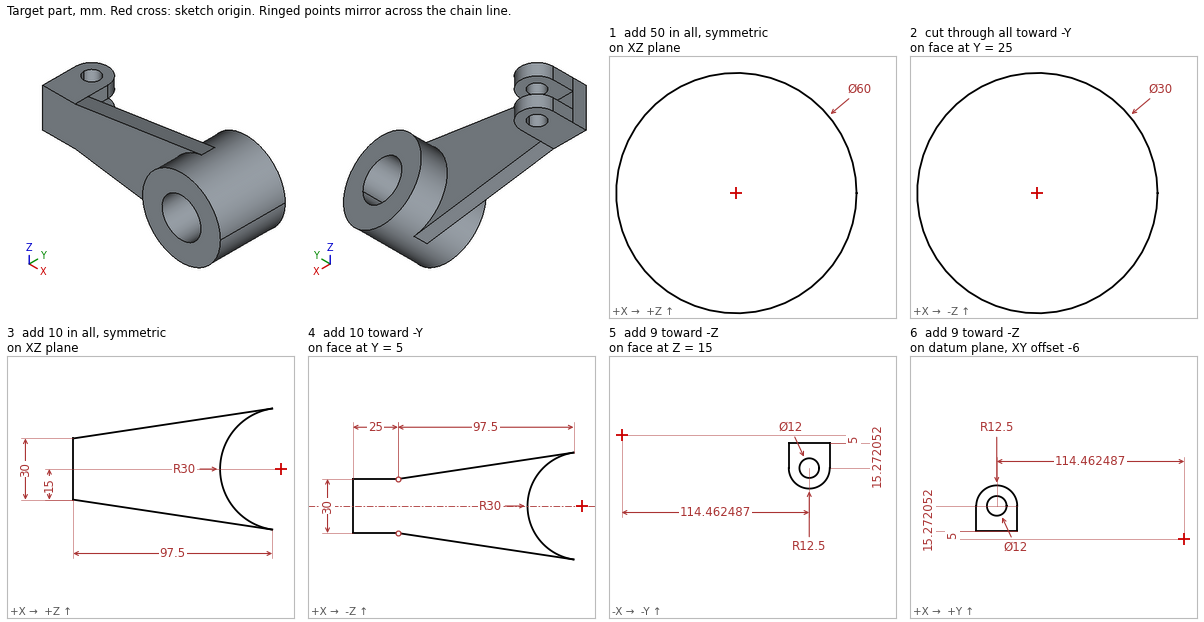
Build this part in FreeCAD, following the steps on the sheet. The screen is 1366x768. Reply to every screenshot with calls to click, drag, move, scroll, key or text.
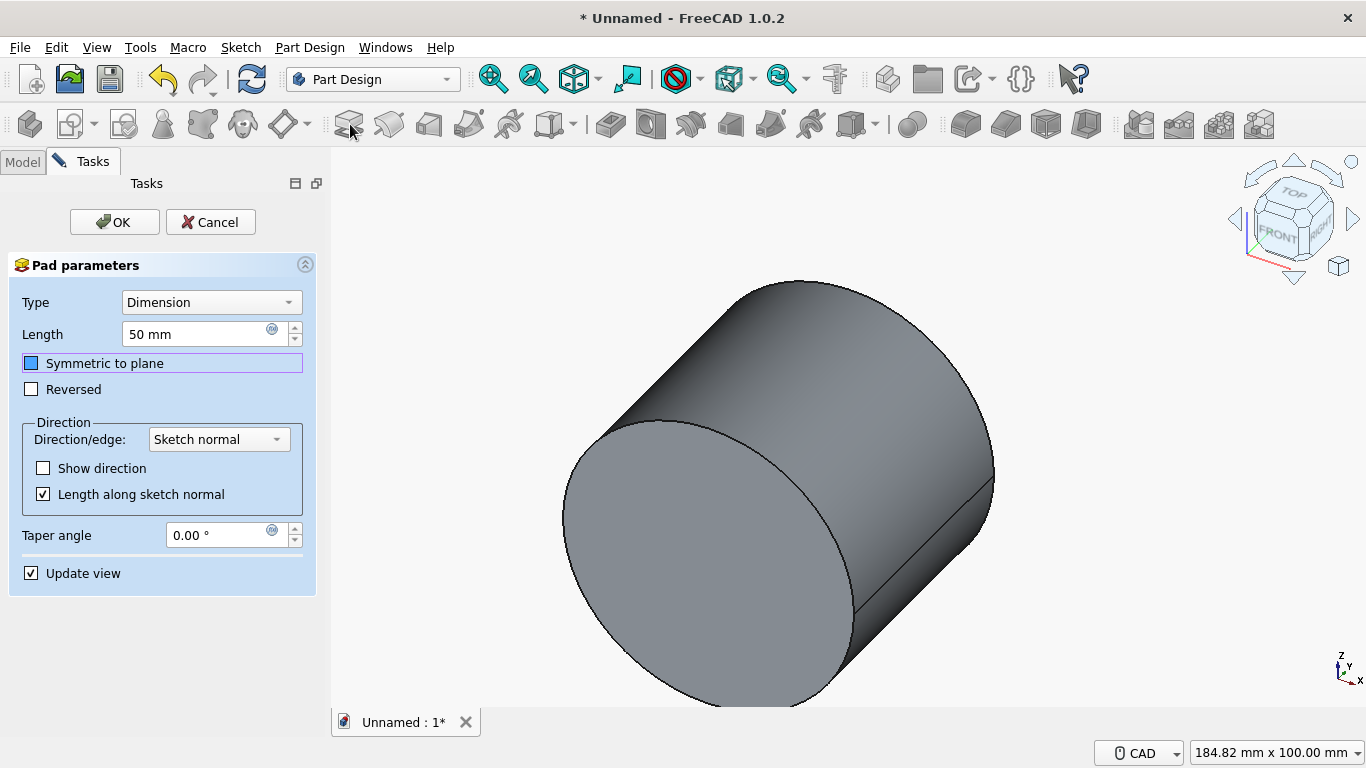
click(30, 363)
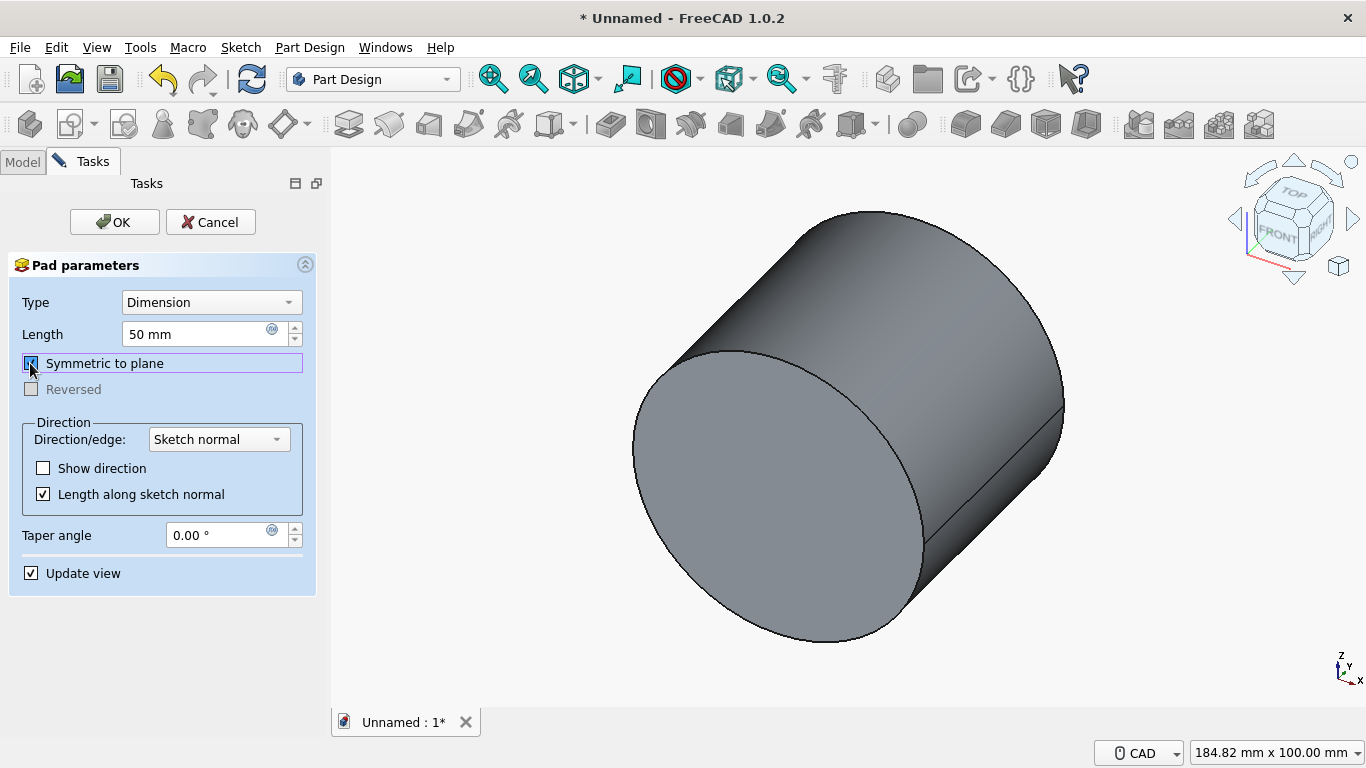
click(115, 222)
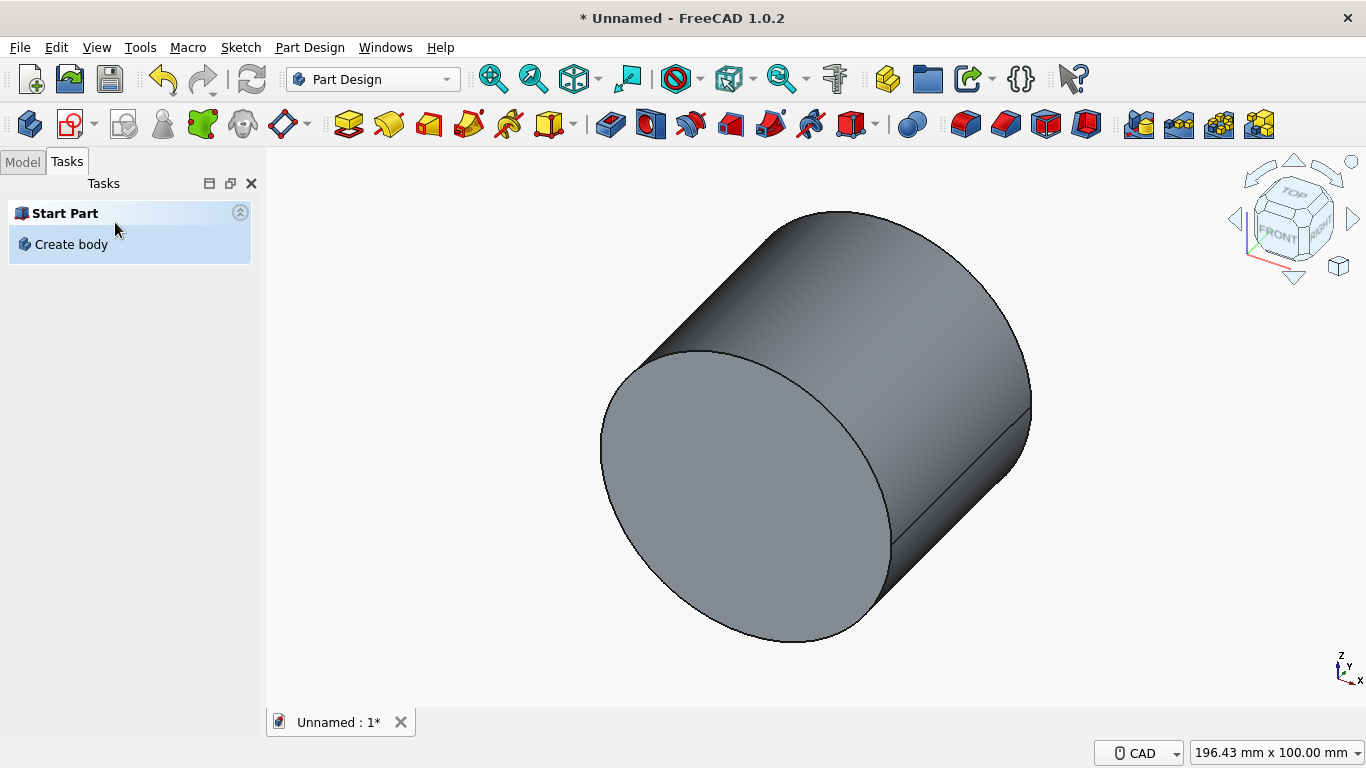
key(4)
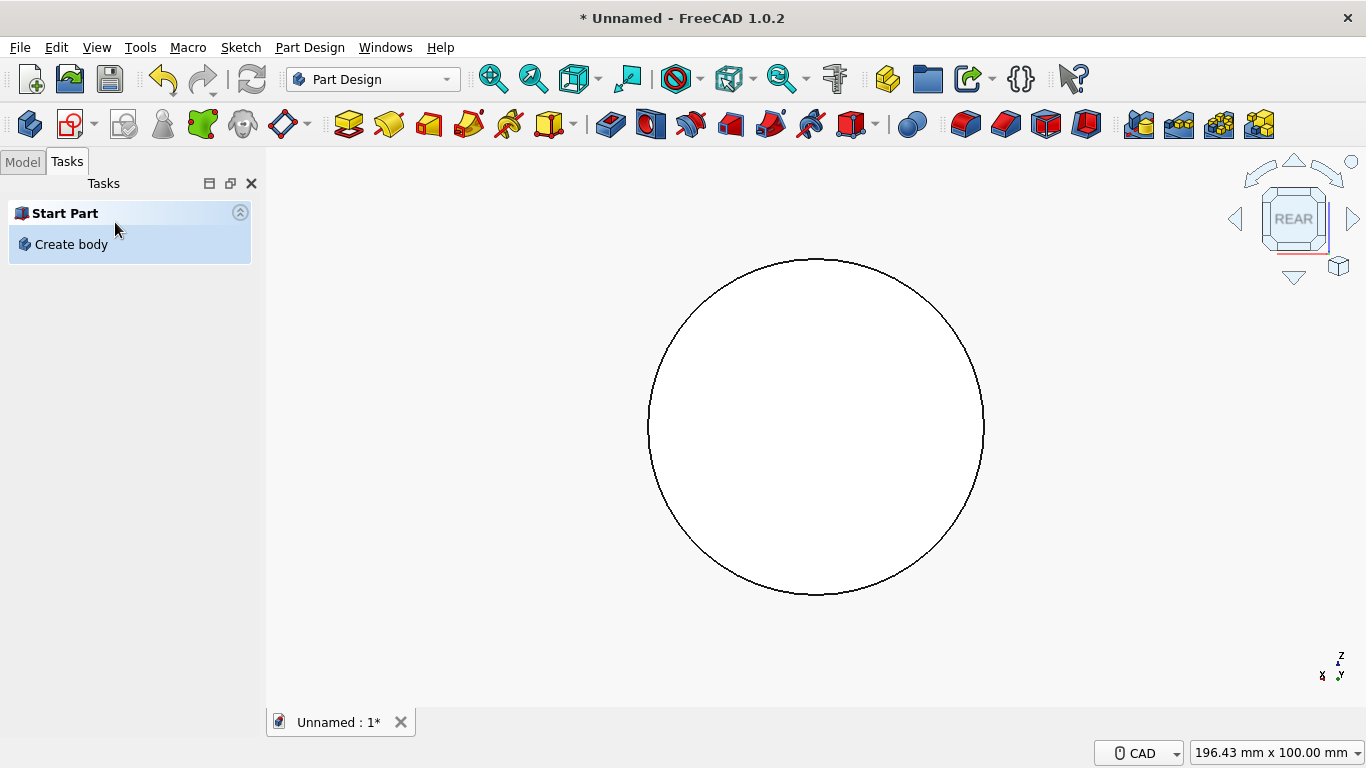
click(816, 426)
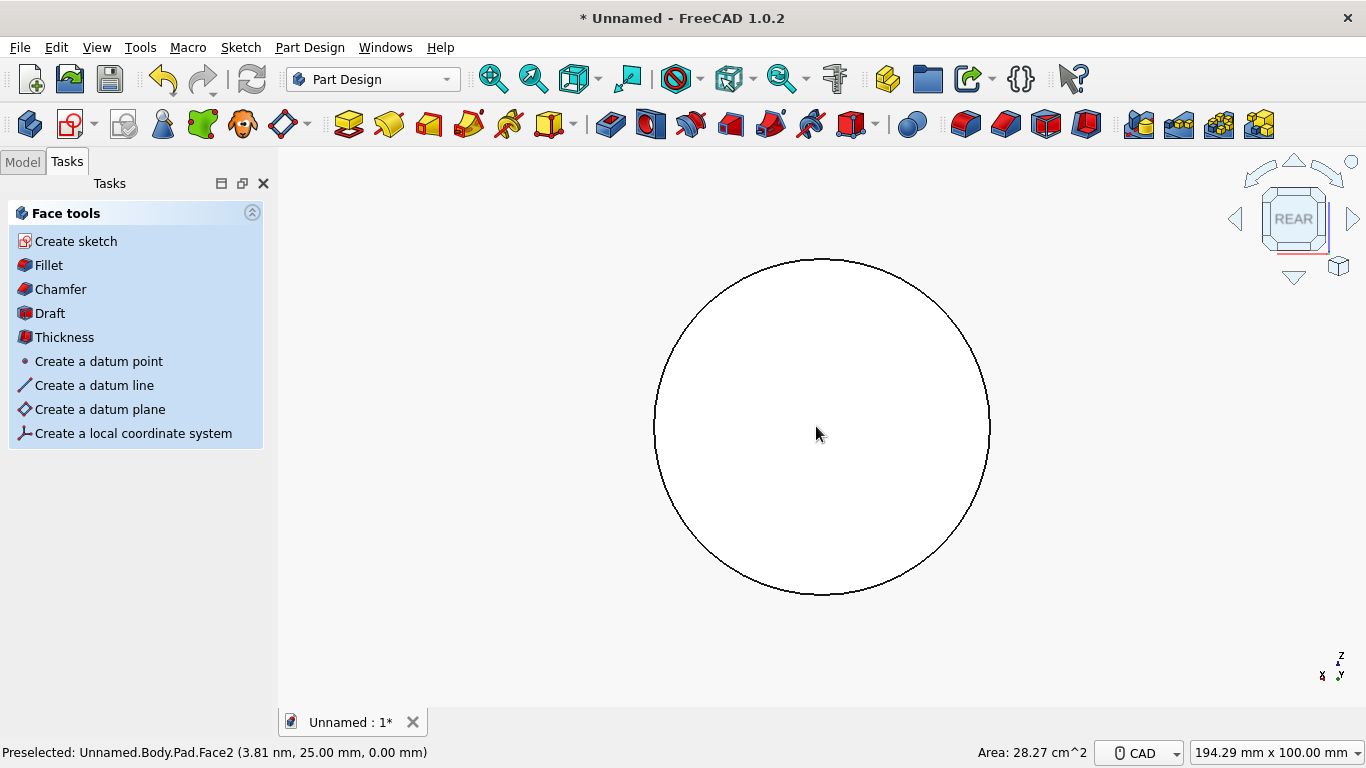
click(70, 124)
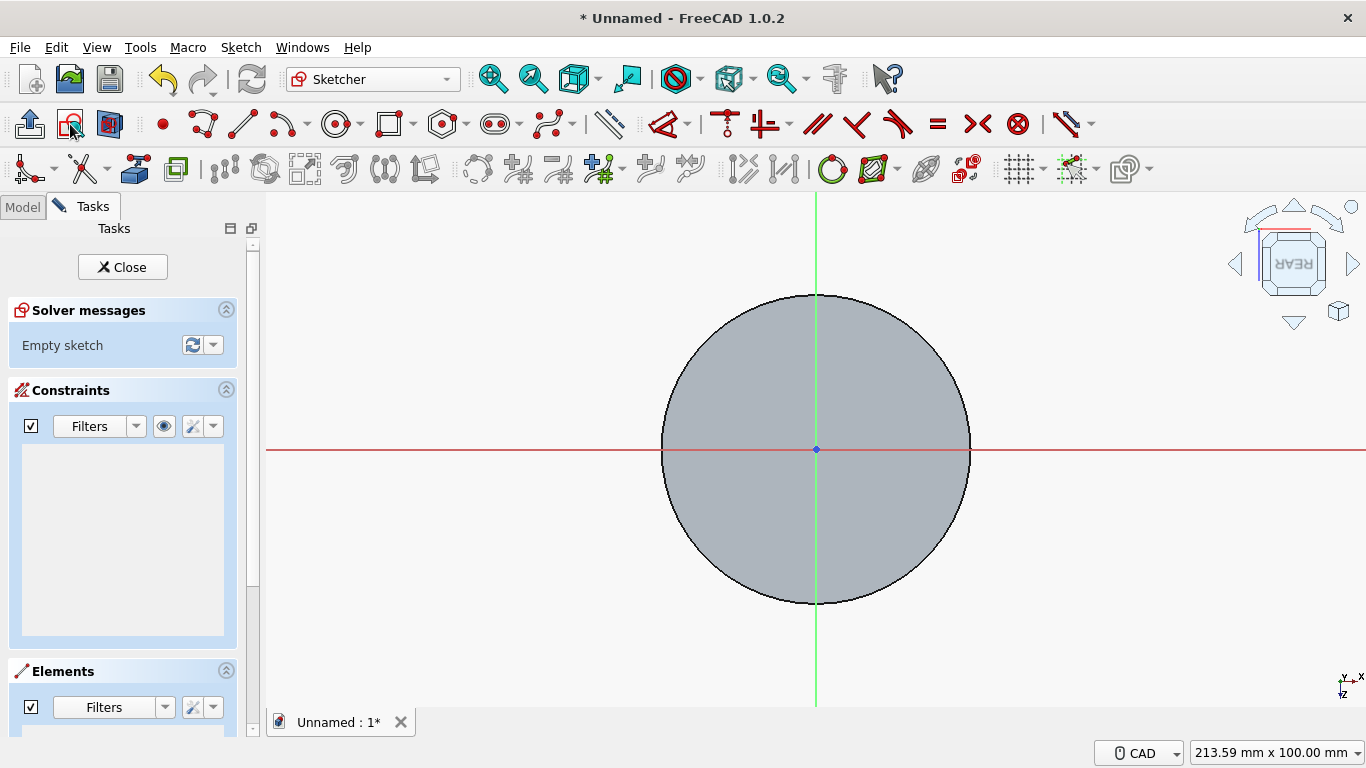
scroll(872, 450, up, 4)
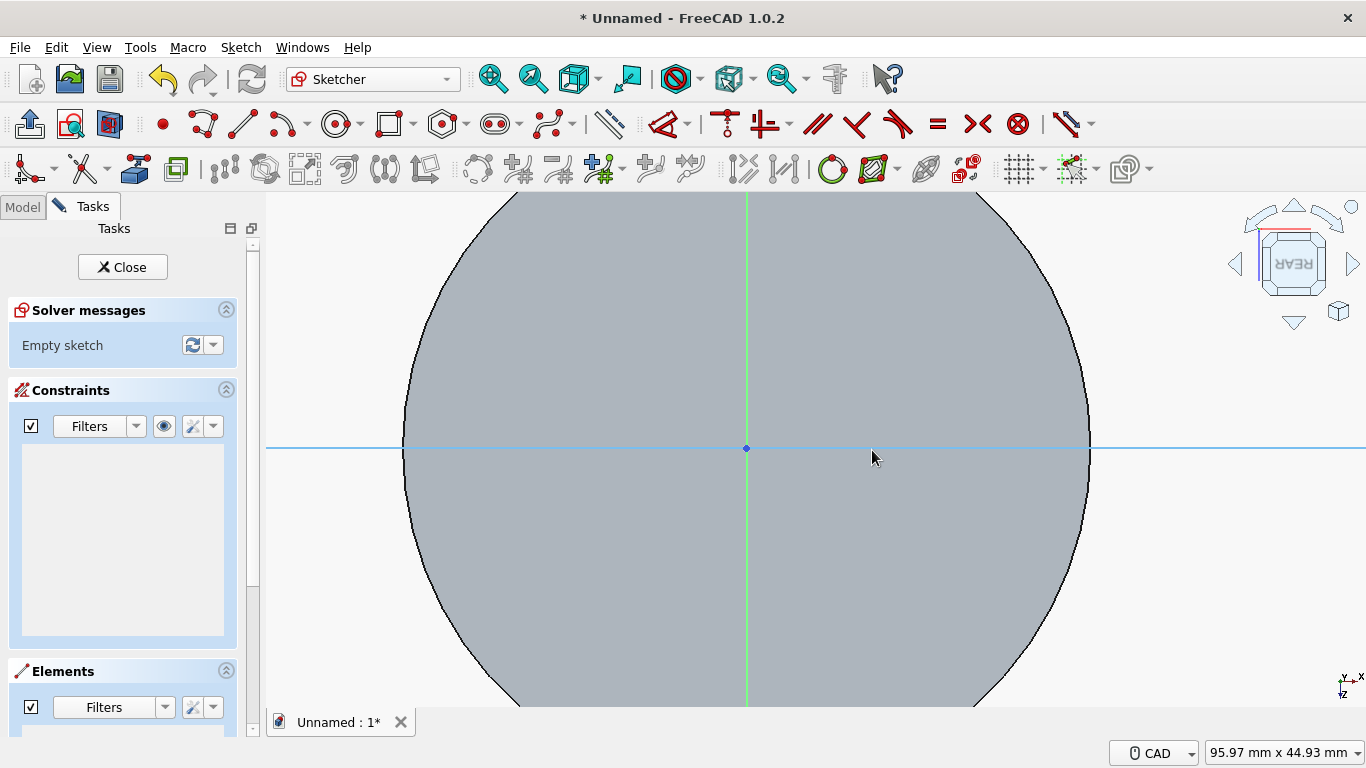
key(g)
key(c)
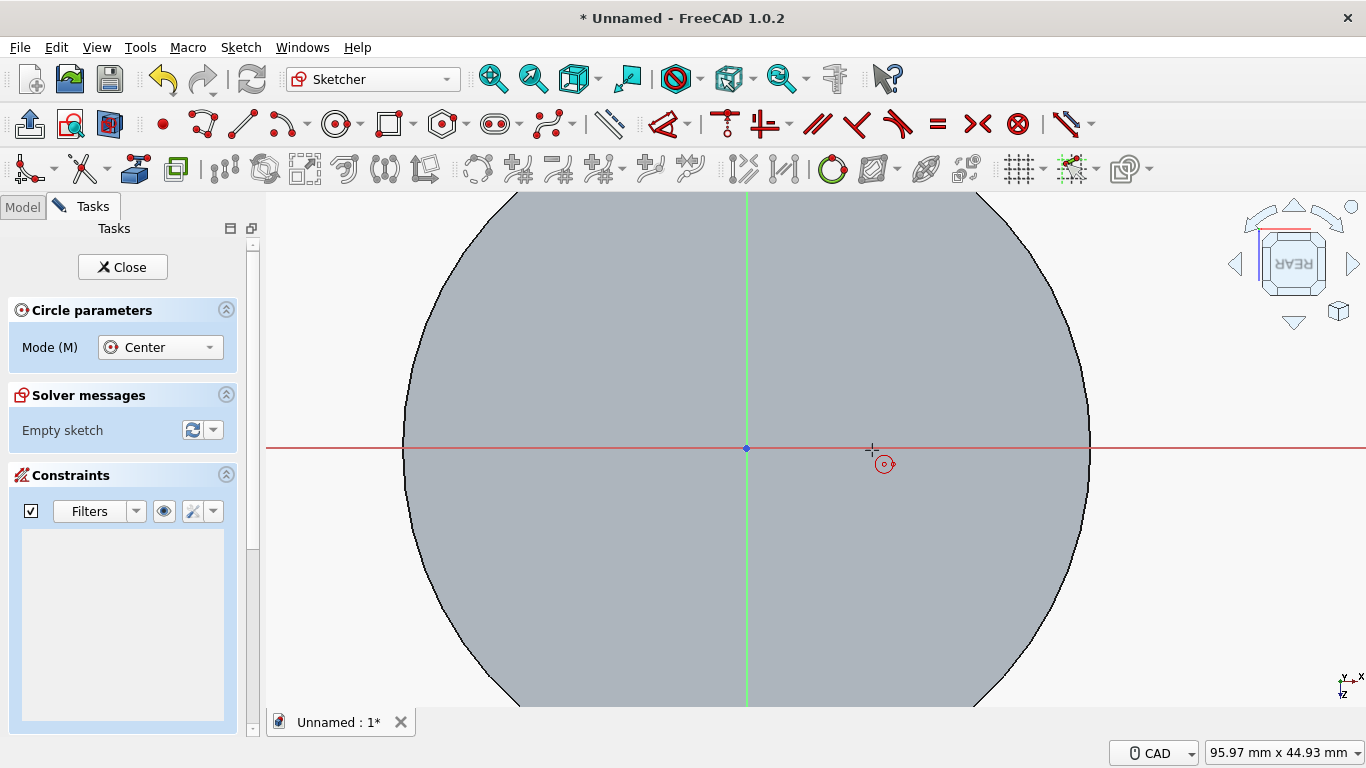
click(747, 448)
move(868, 327)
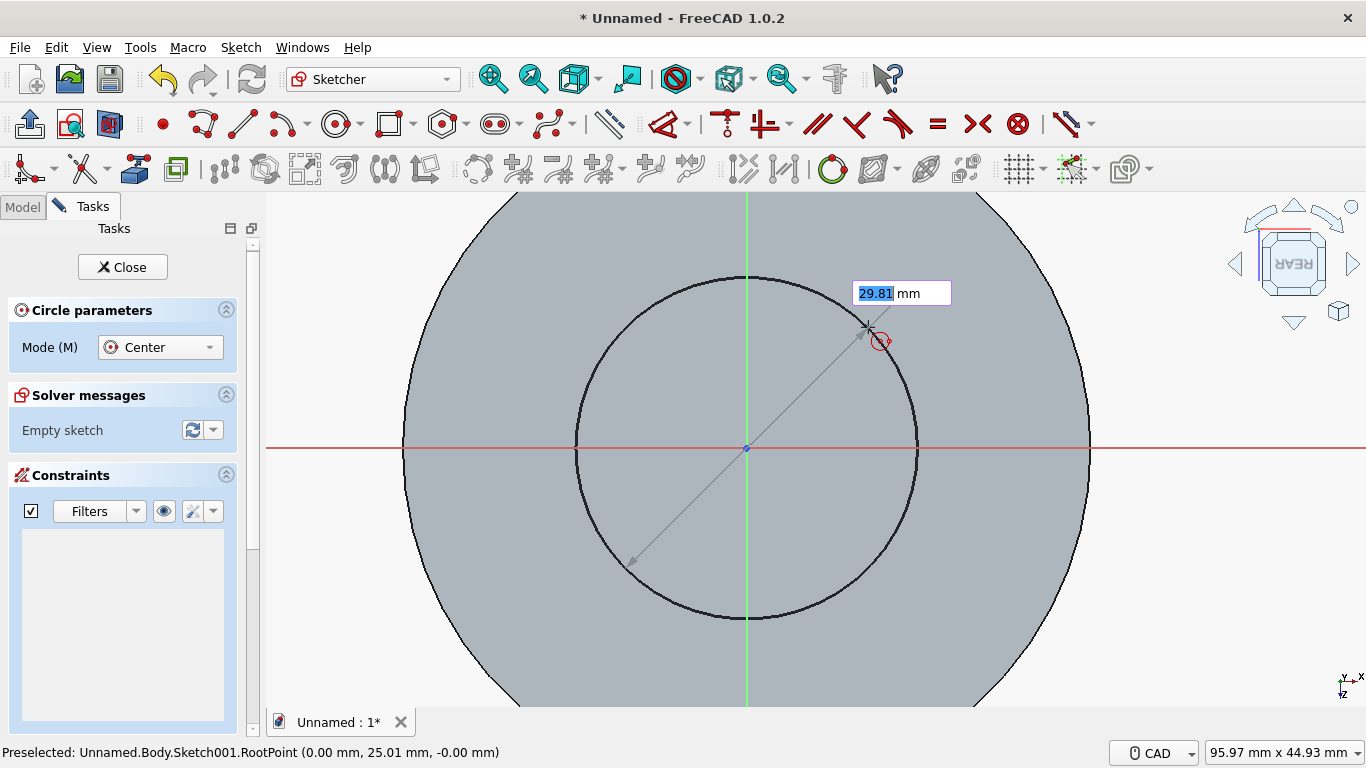
text(30)
key(Return)
key(Escape)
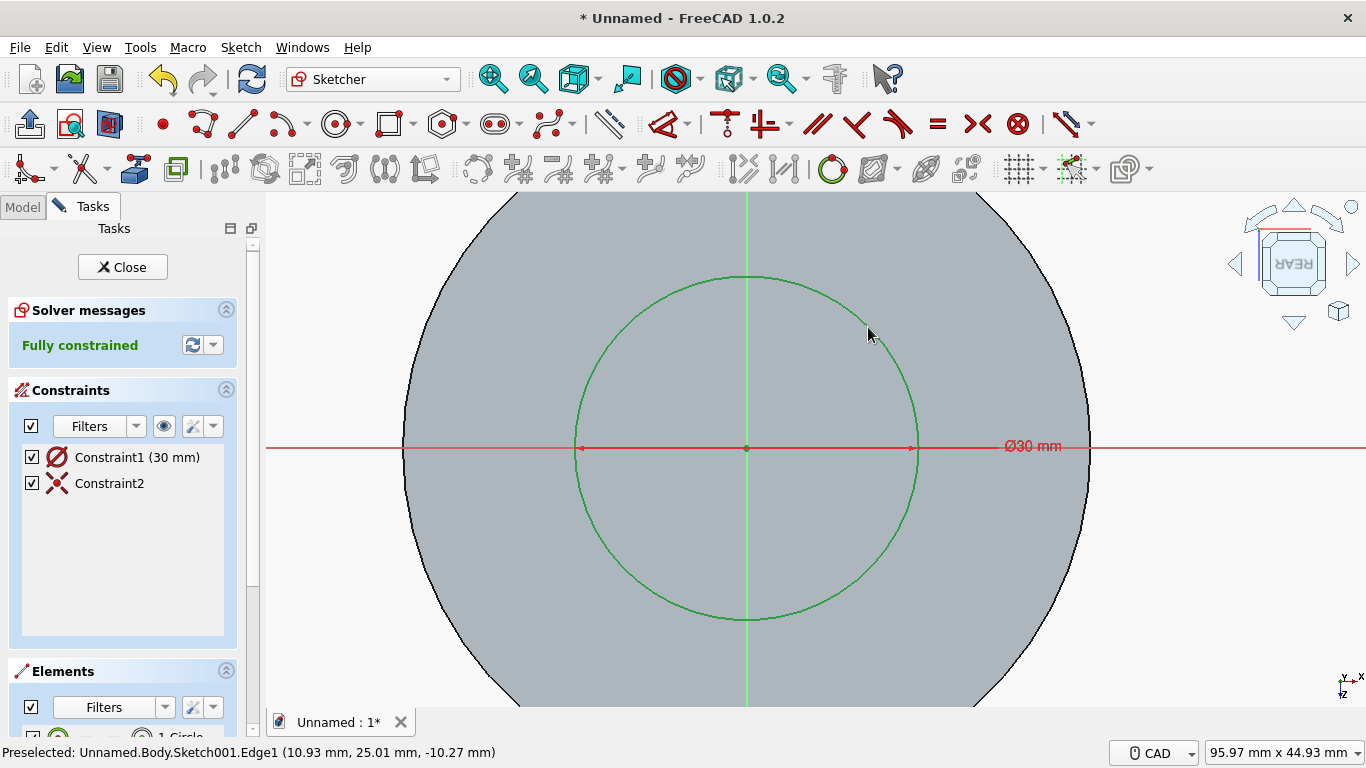
click(123, 267)